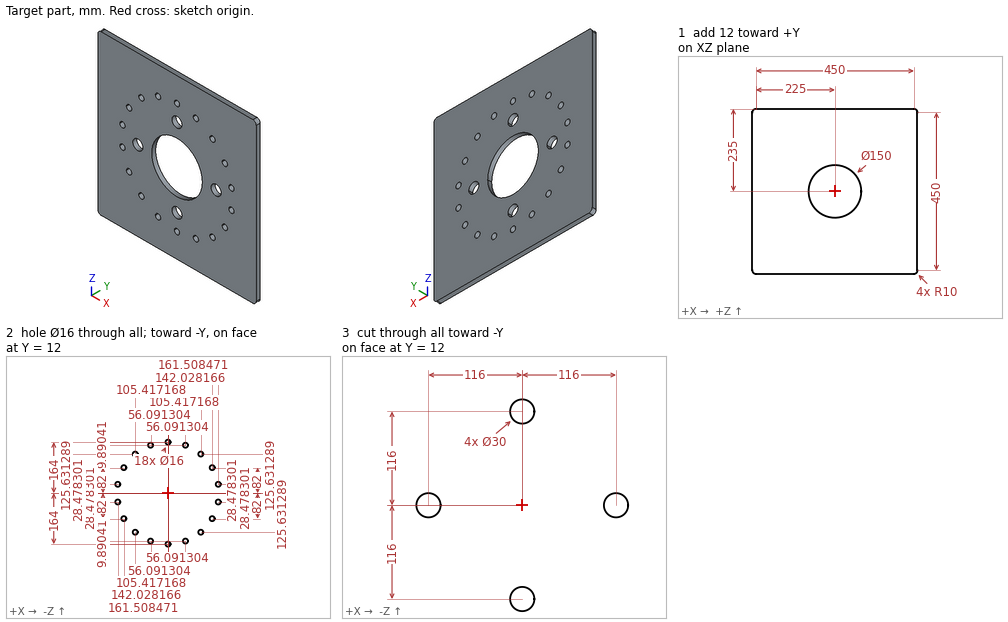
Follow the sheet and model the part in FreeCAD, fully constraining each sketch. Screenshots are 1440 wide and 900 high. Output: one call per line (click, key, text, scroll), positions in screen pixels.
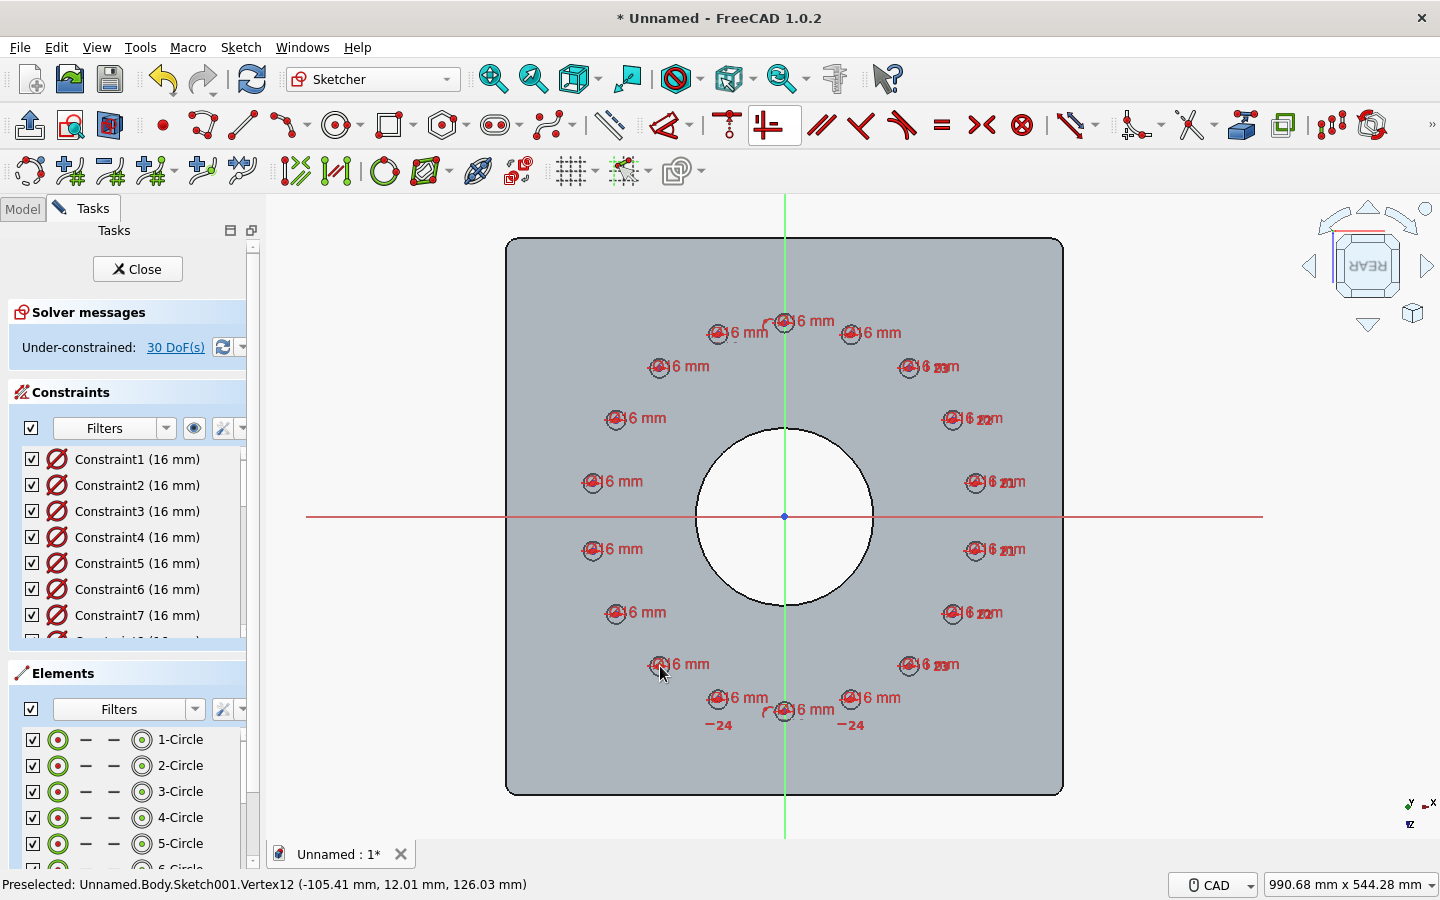
key(h)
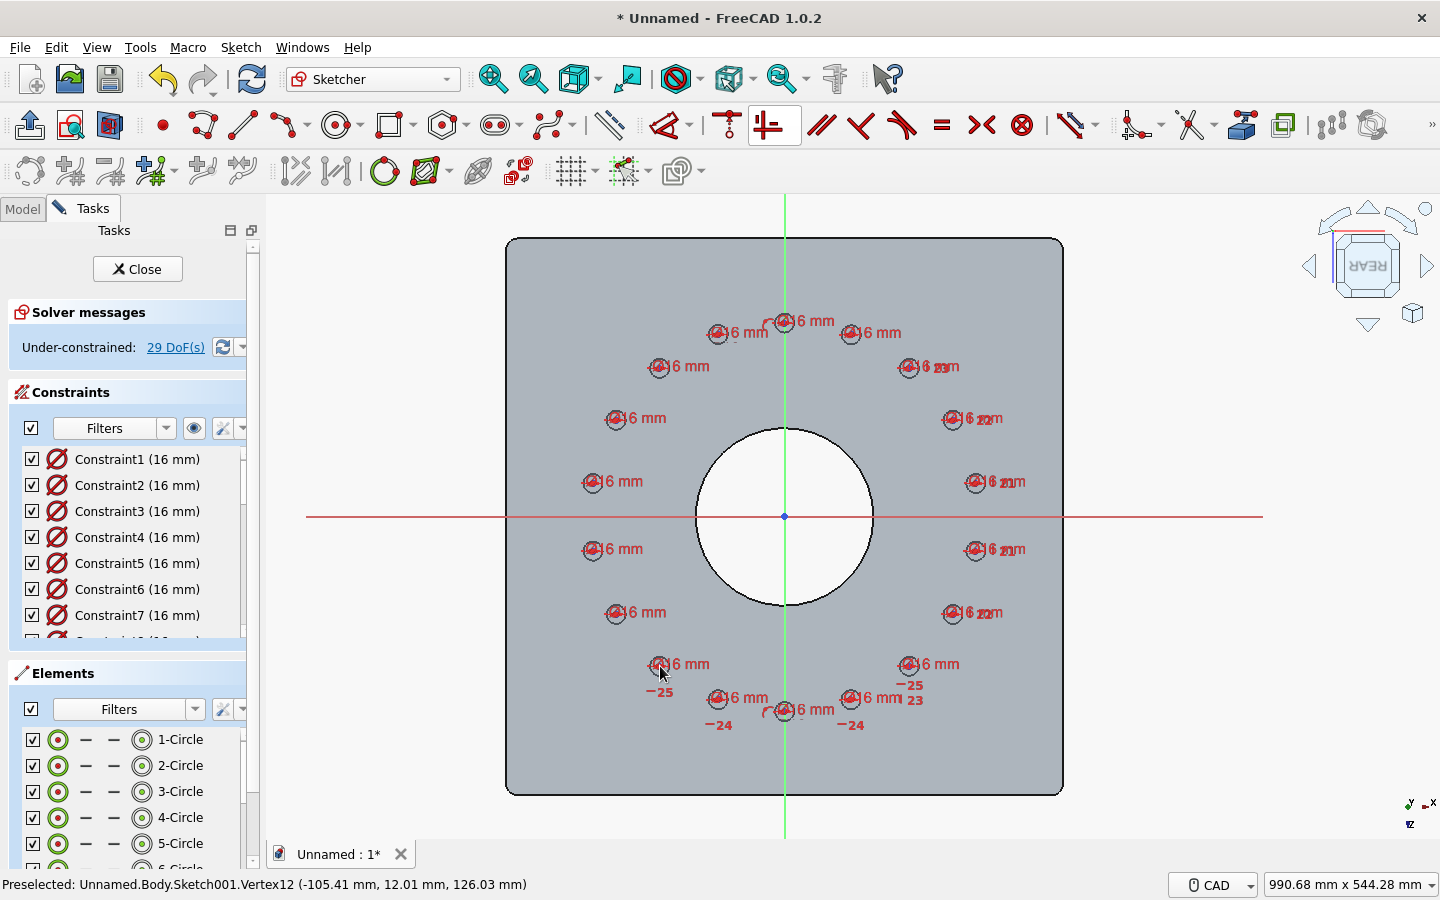
click(593, 551)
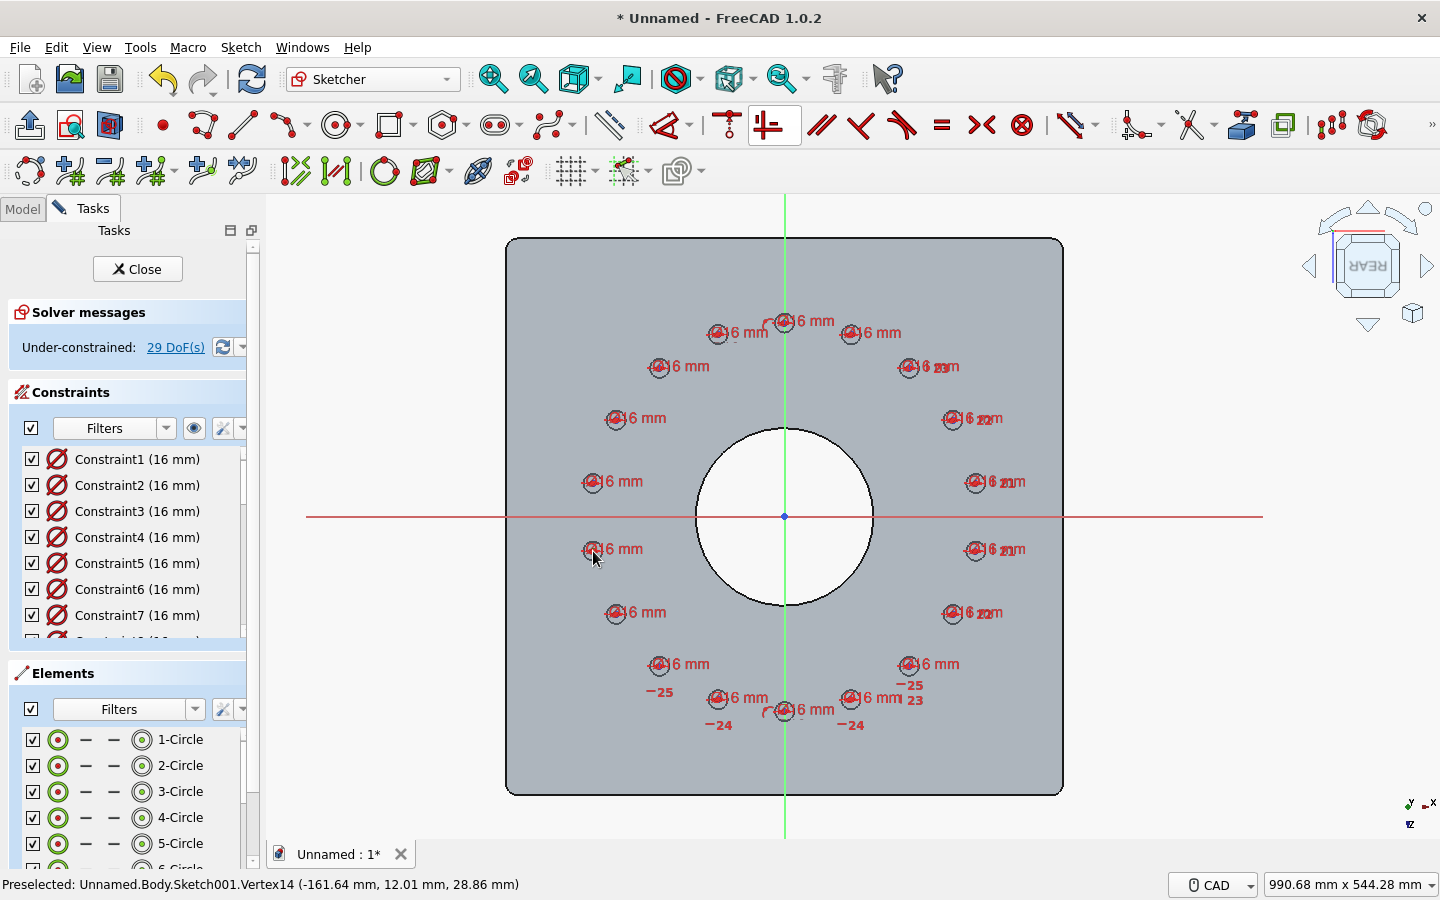
click(593, 483)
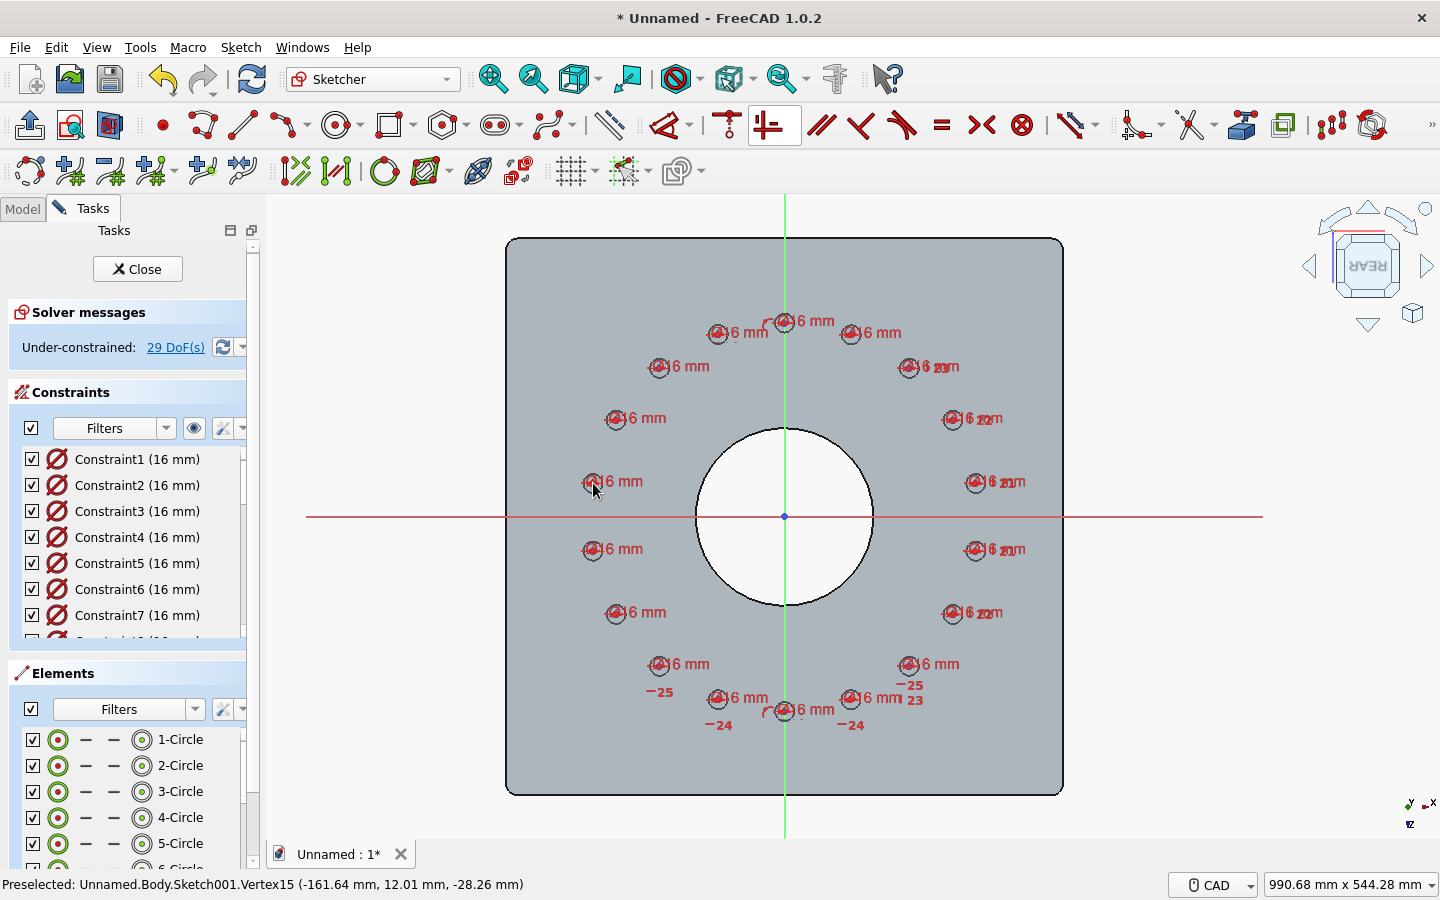
click(796, 126)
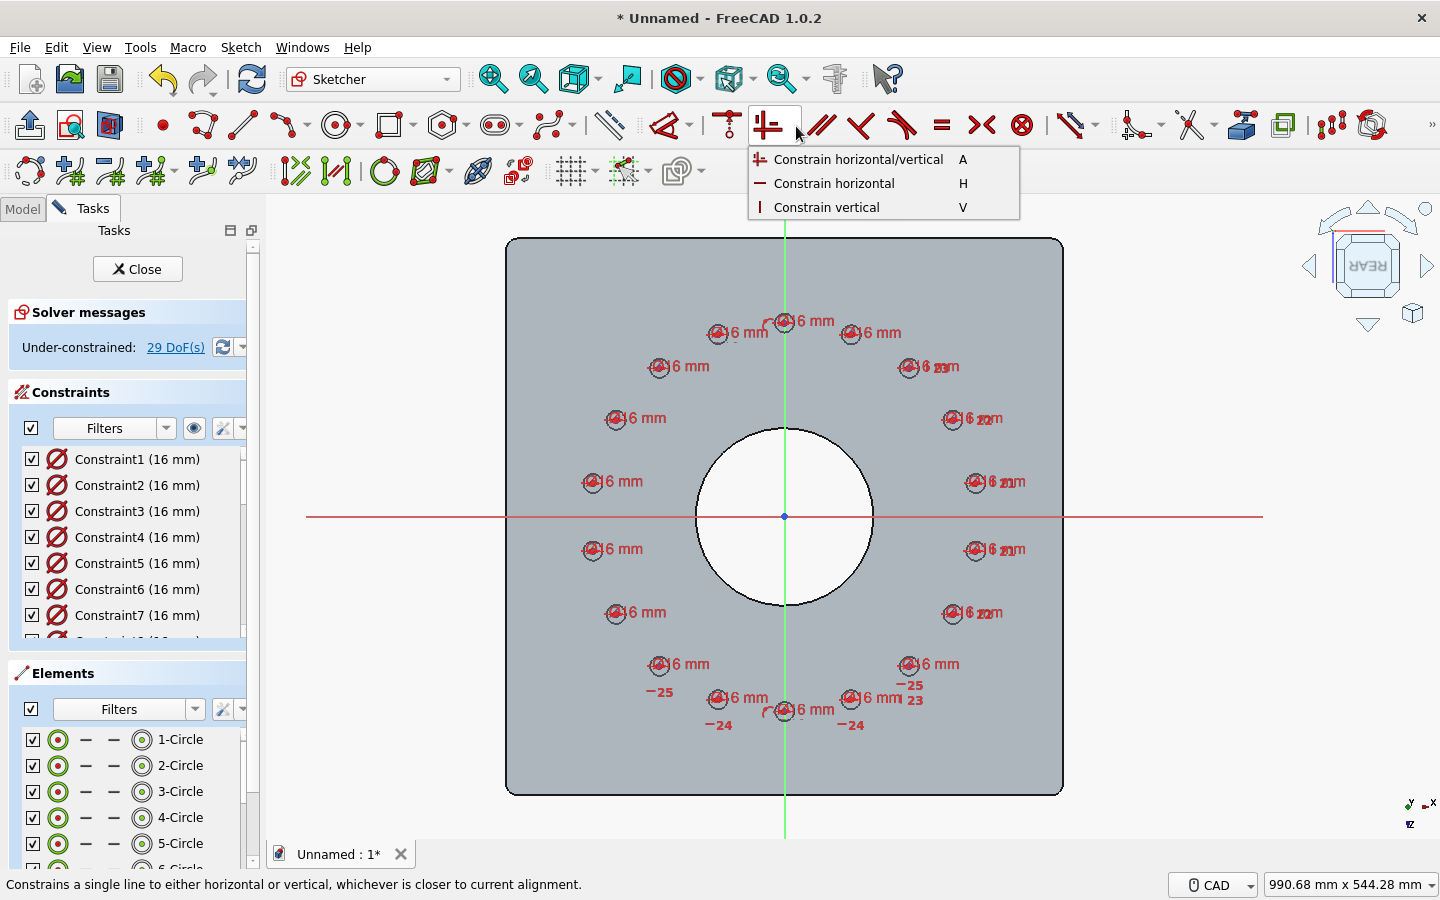
click(884, 207)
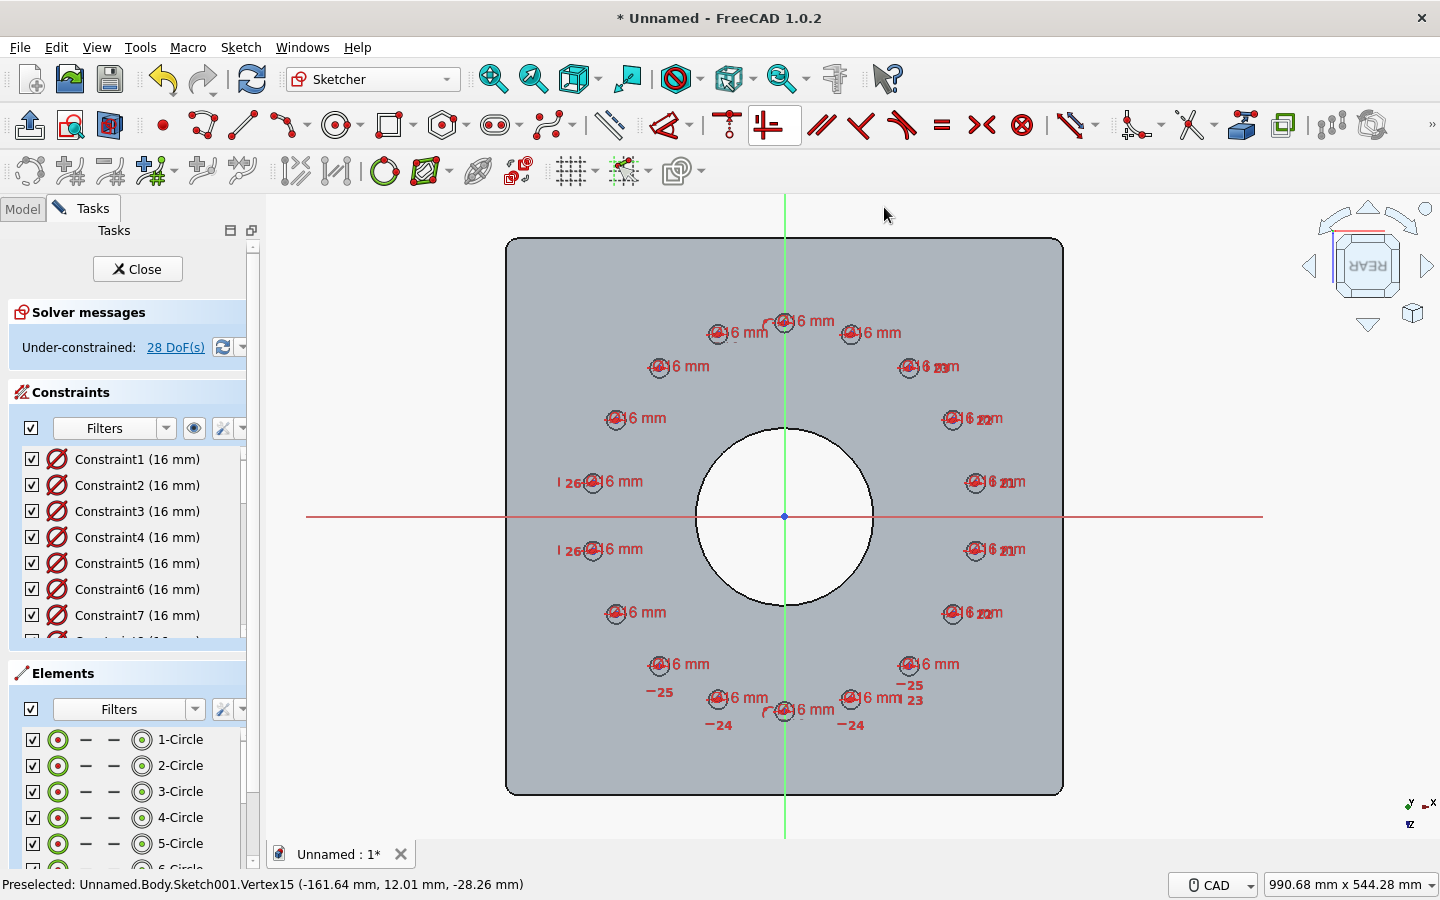
click(616, 614)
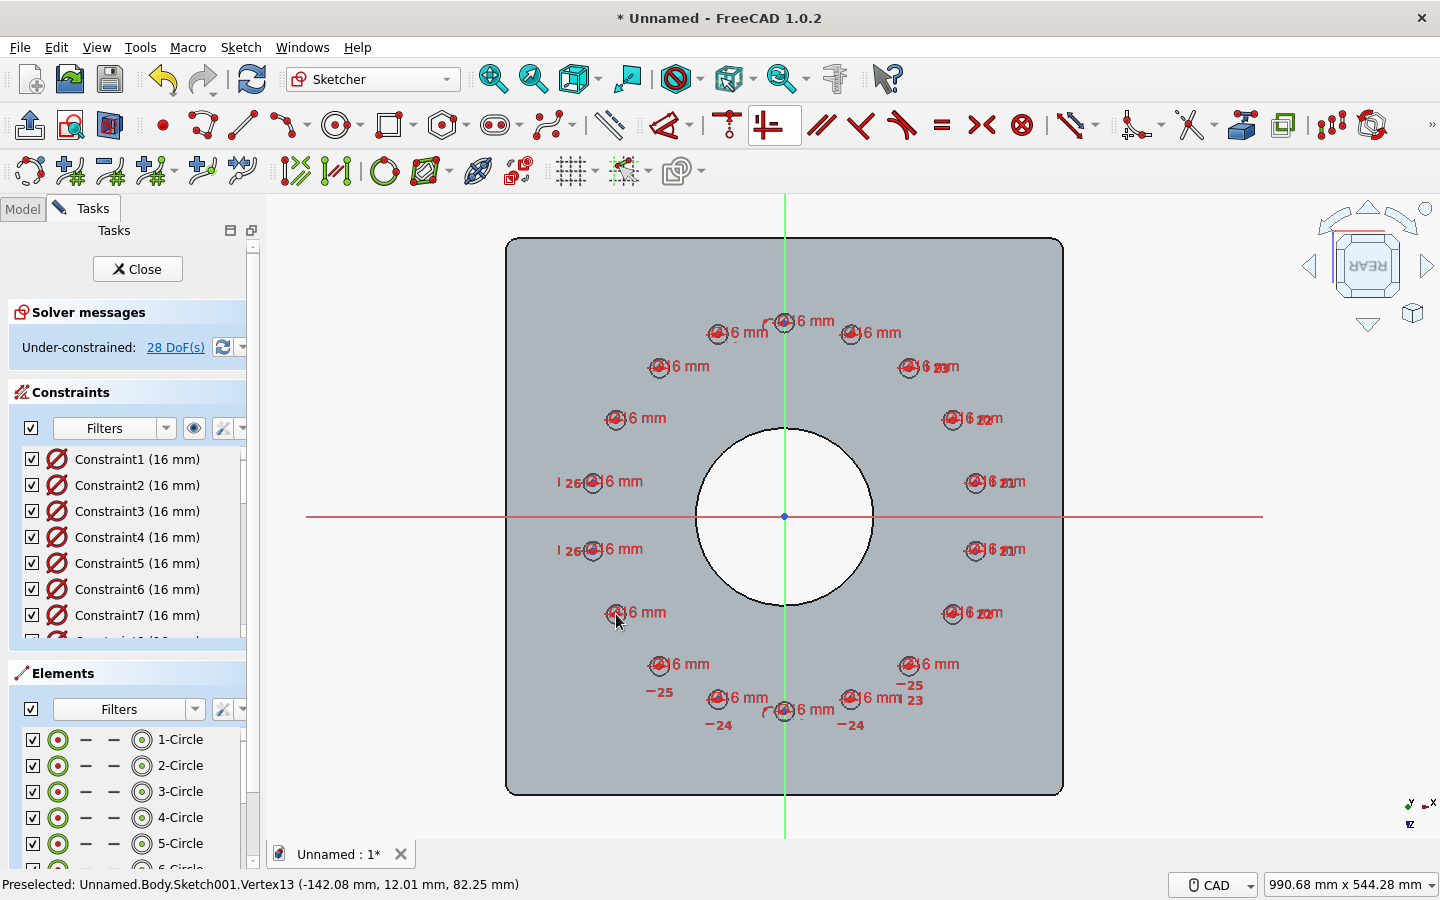
click(616, 420)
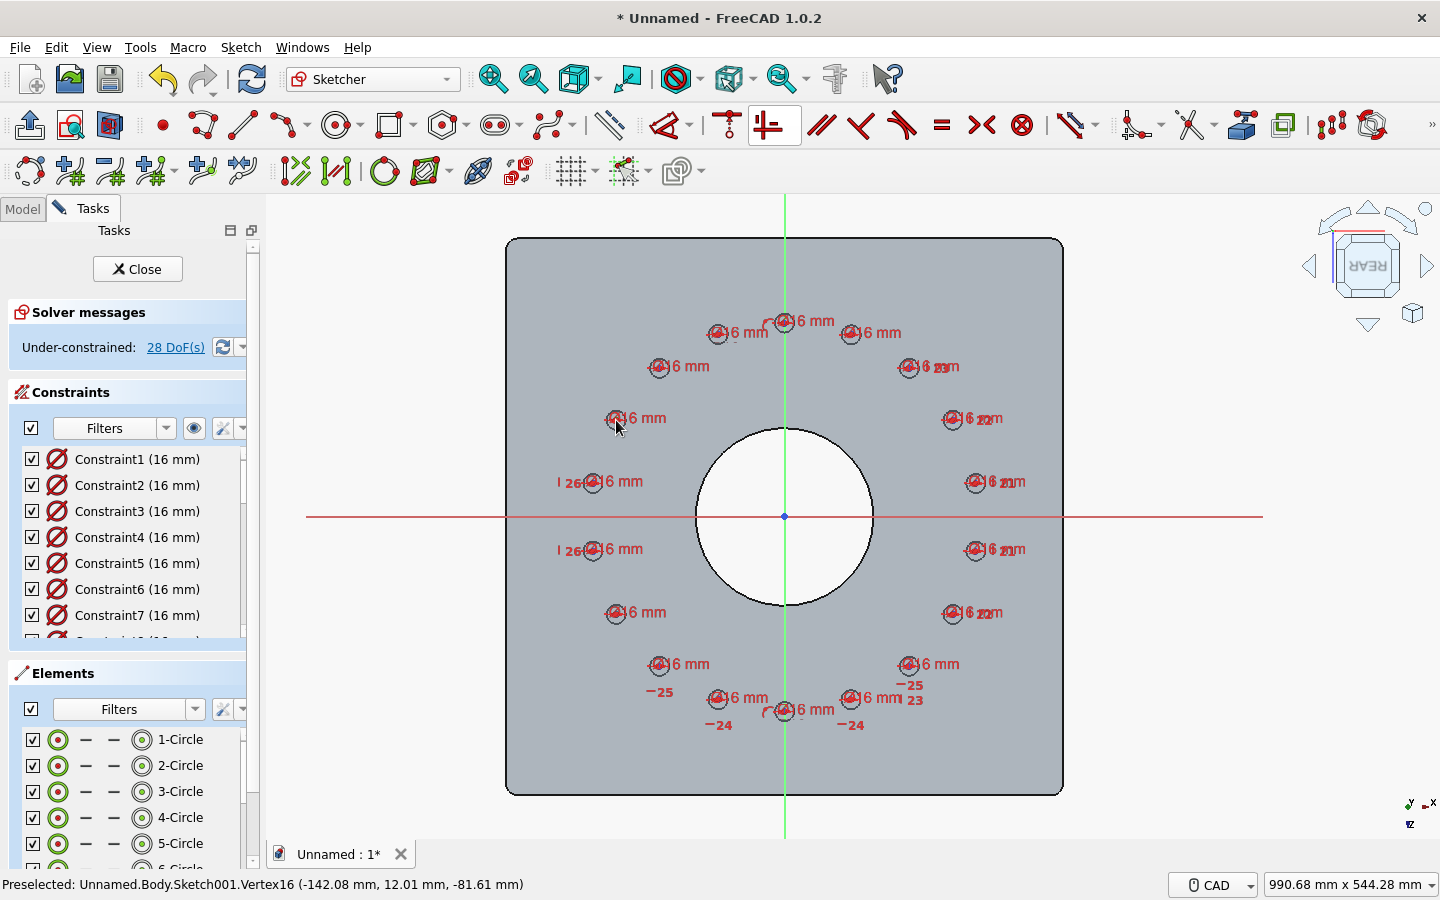
click(796, 126)